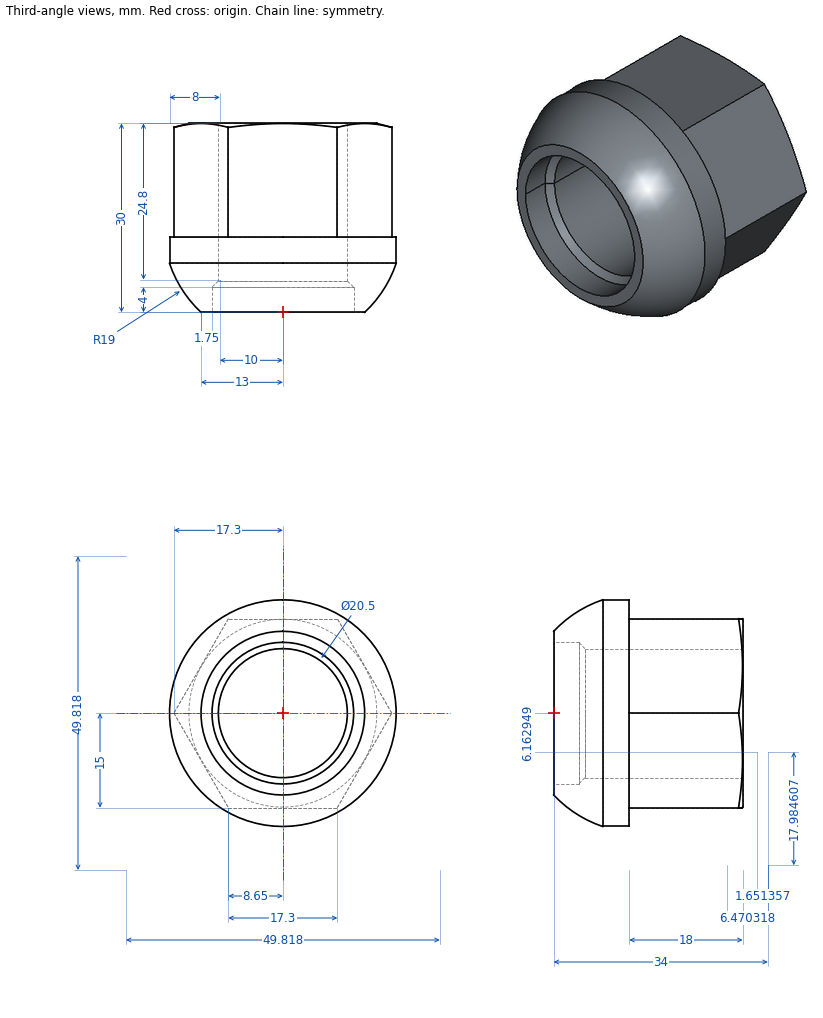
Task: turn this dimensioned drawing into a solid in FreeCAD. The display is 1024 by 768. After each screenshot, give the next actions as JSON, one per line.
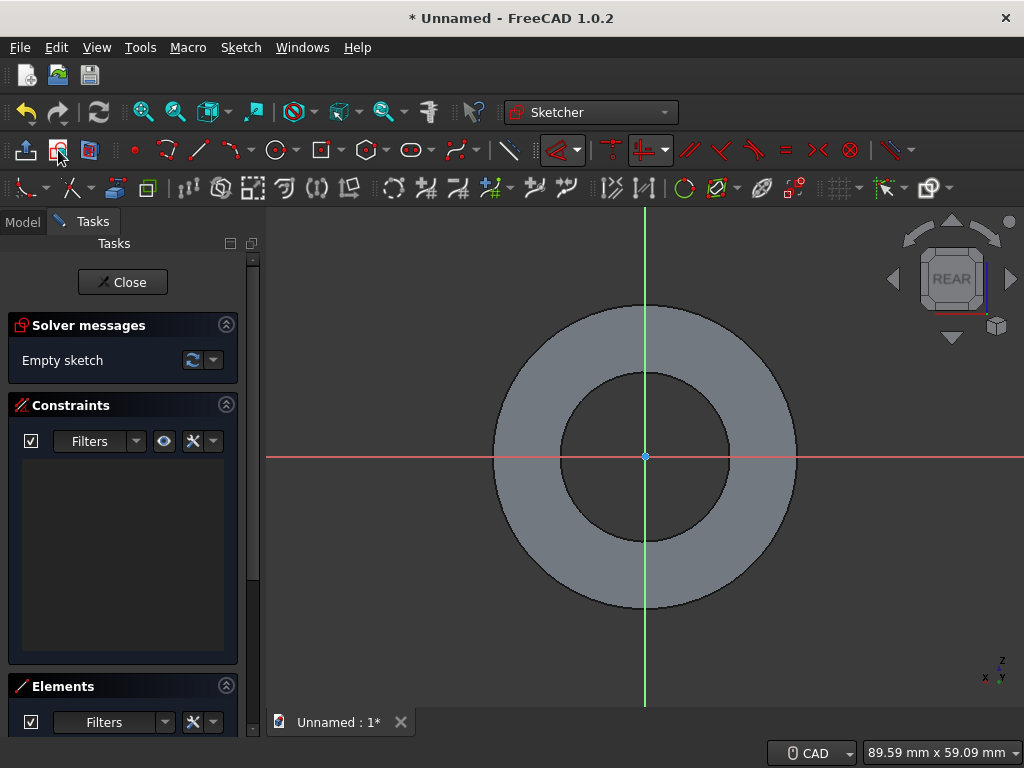
{"action": "scroll", "coordinate": [728, 457], "scroll_direction": "up", "scroll_amount": 3}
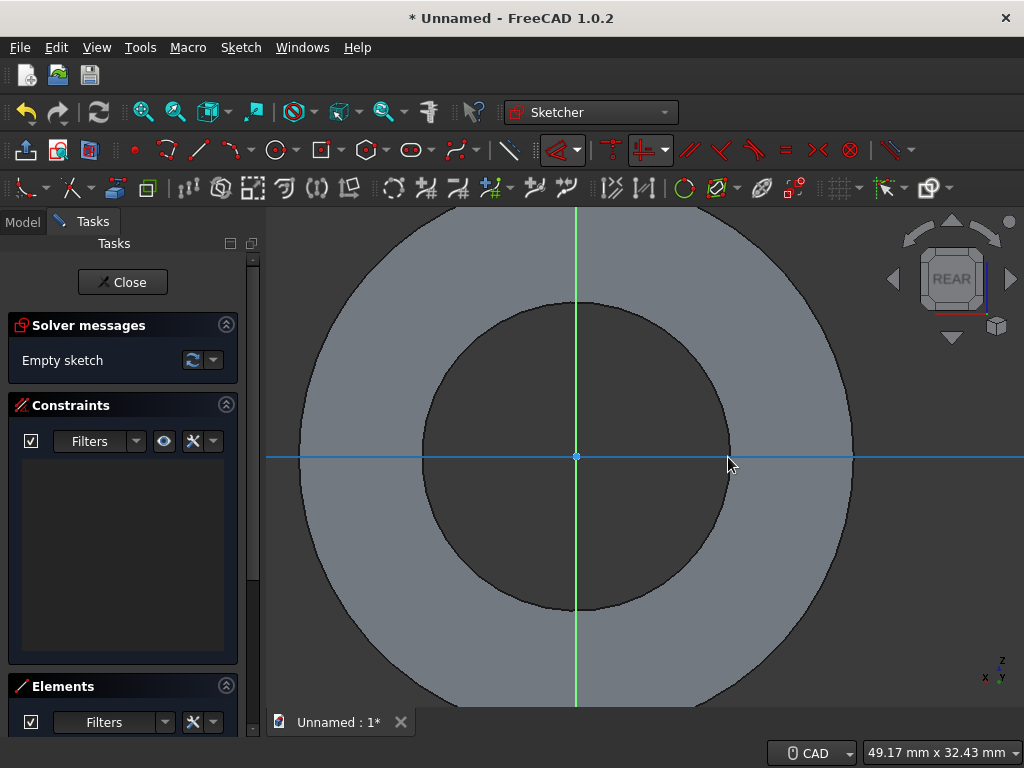
{"action": "key", "text": "g c"}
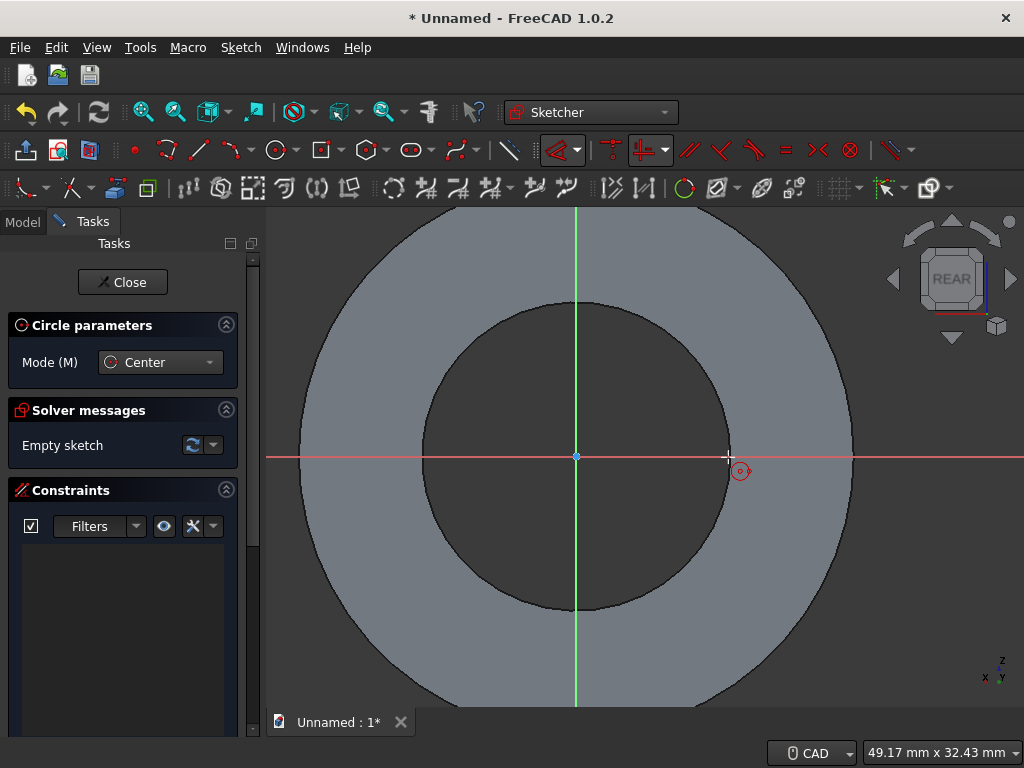
{"action": "left_click", "coordinate": [576, 457]}
{"action": "left_click", "coordinate": [688, 345]}
{"action": "key", "text": "Escape"}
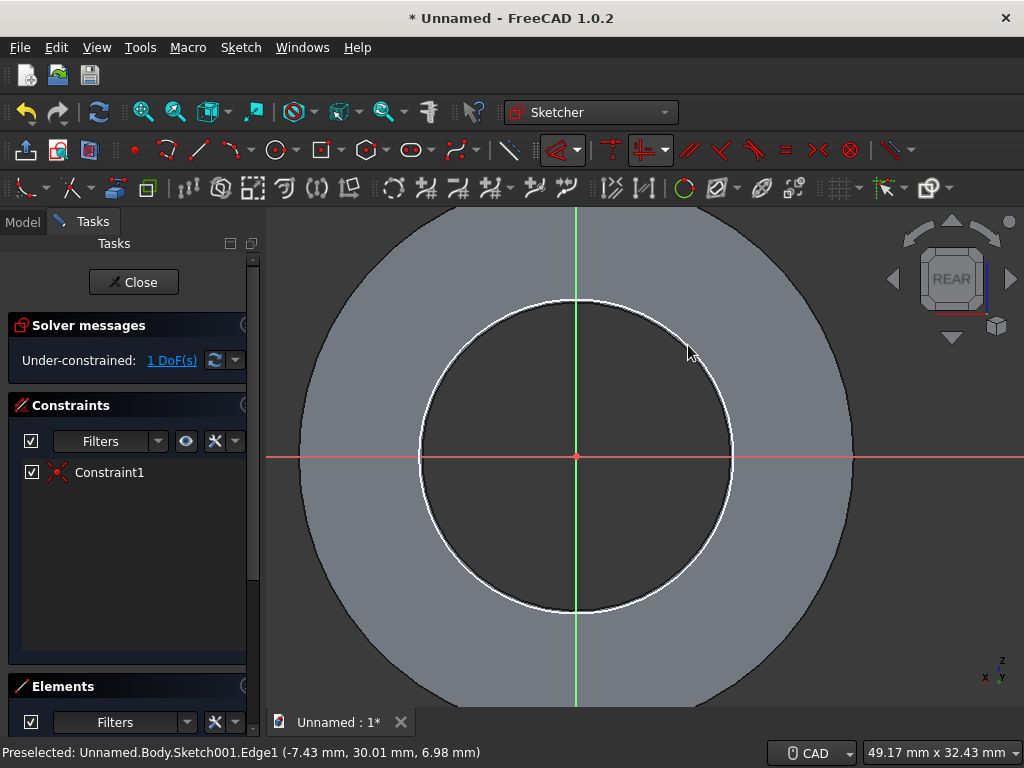
{"action": "left_click", "coordinate": [687, 345]}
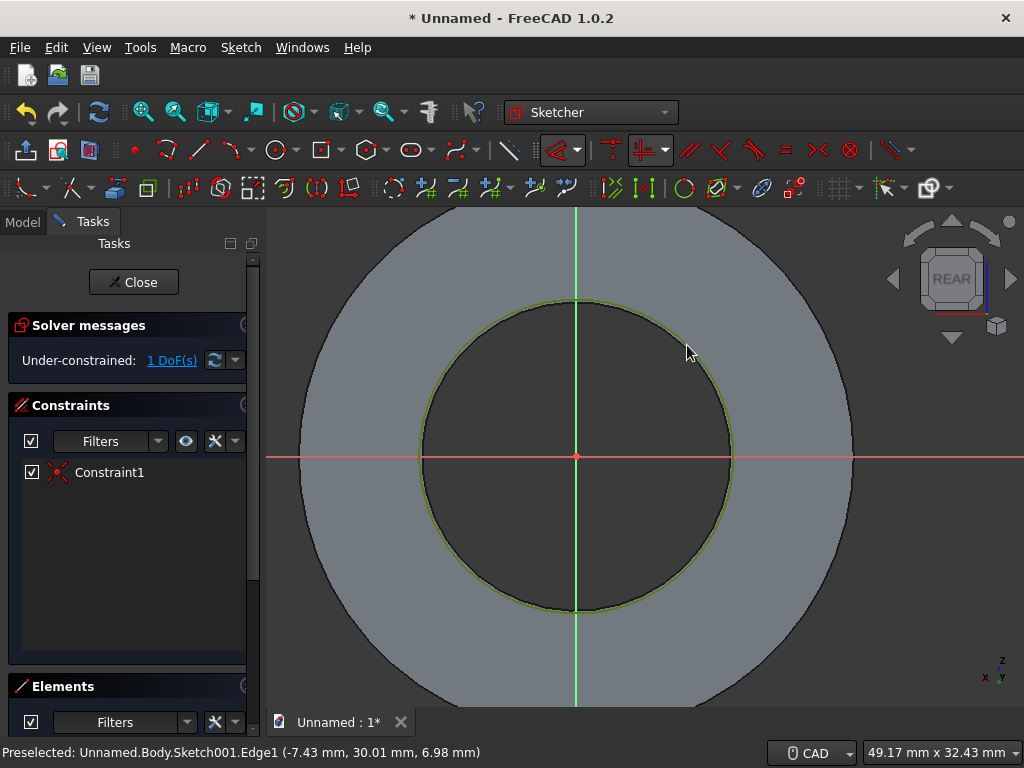
{"action": "key", "text": "k o"}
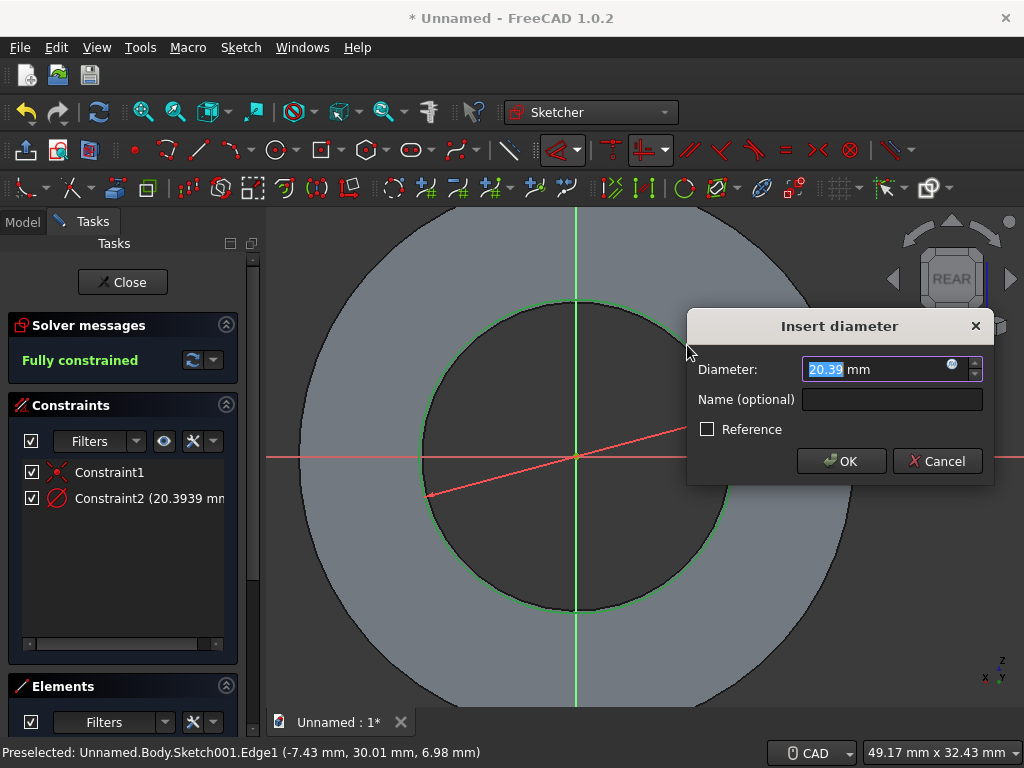
{"action": "type", "text": "20.5"}
{"action": "key", "text": "Return"}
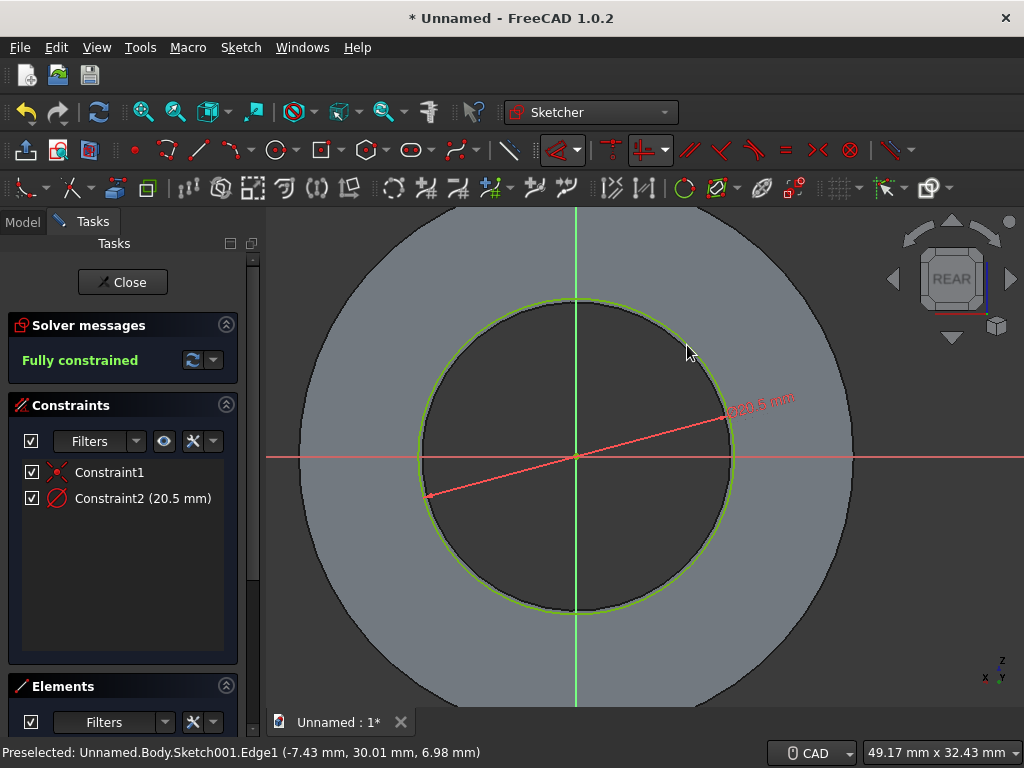
{"action": "left_click", "coordinate": [123, 282]}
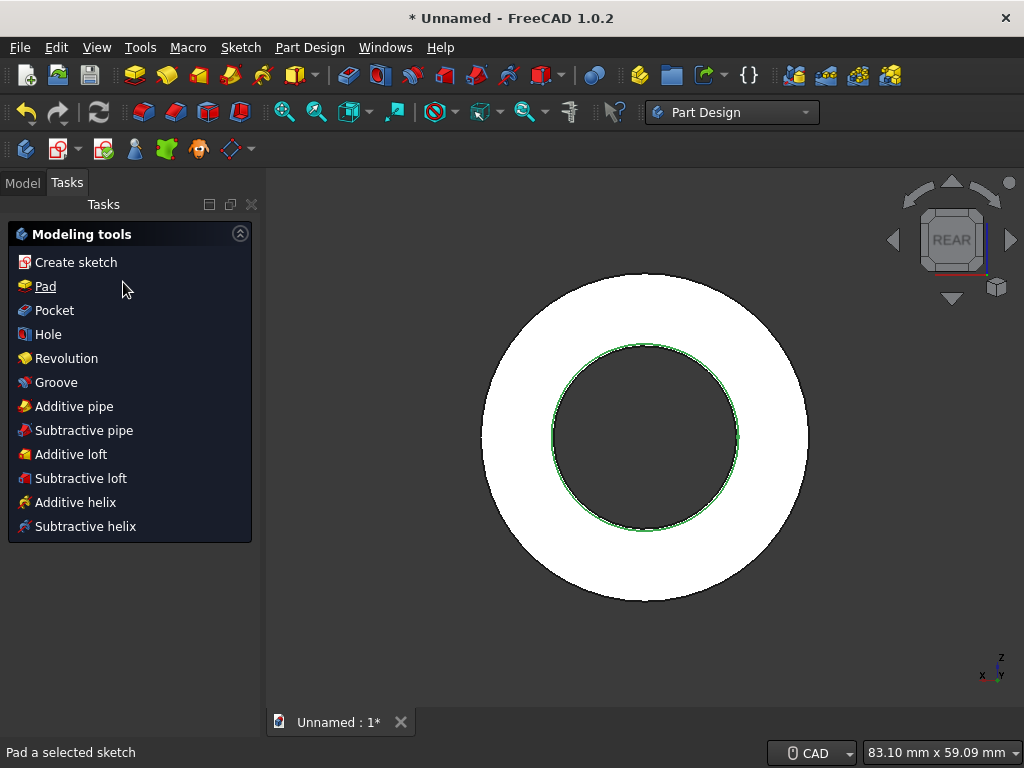
{"action": "left_click", "coordinate": [350, 76]}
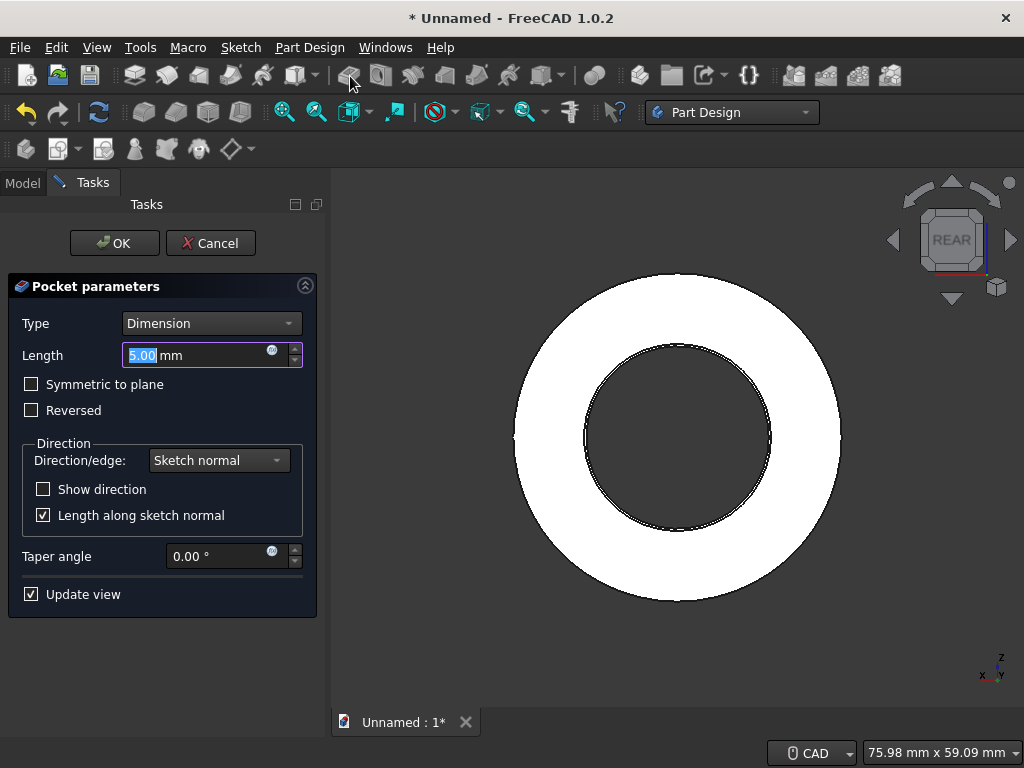
{"action": "left_click", "coordinate": [212, 324]}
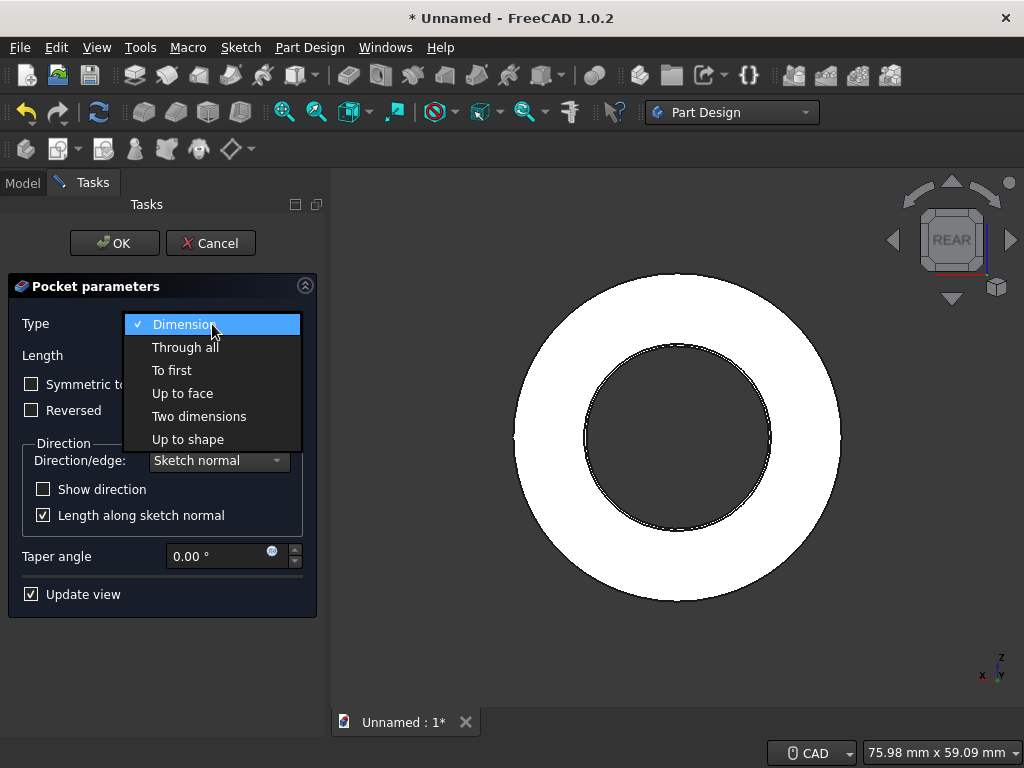
{"action": "left_click", "coordinate": [212, 348]}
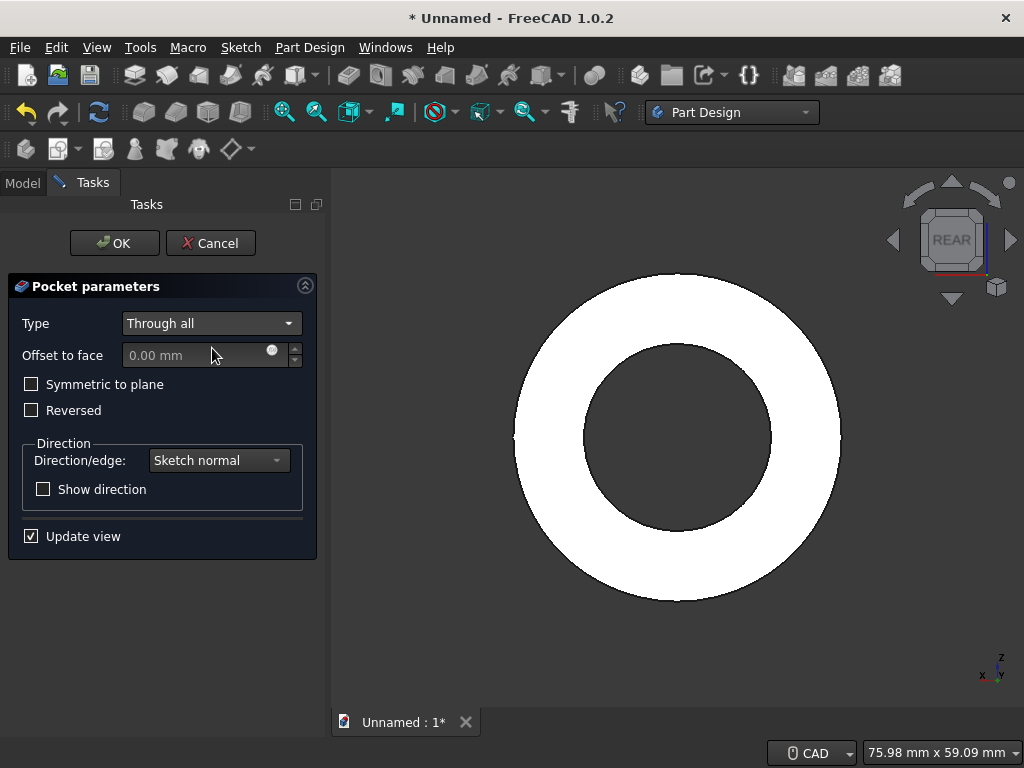
{"action": "left_click", "coordinate": [115, 243]}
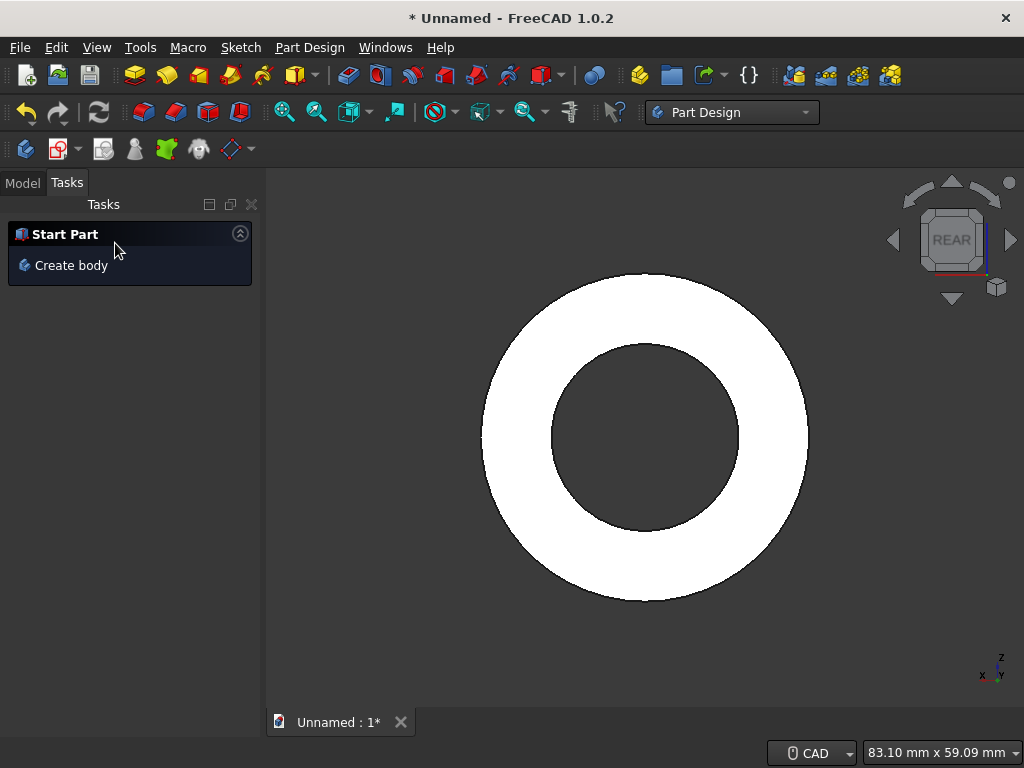
{"action": "left_click", "coordinate": [551, 530]}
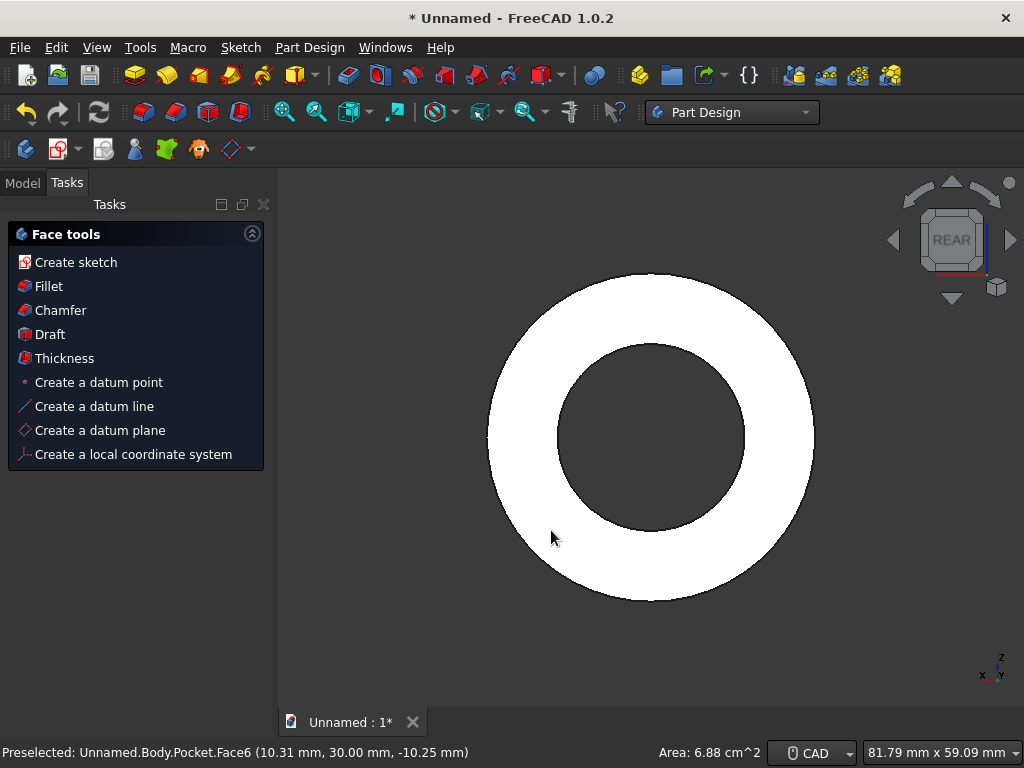
{"action": "left_click", "coordinate": [58, 150]}